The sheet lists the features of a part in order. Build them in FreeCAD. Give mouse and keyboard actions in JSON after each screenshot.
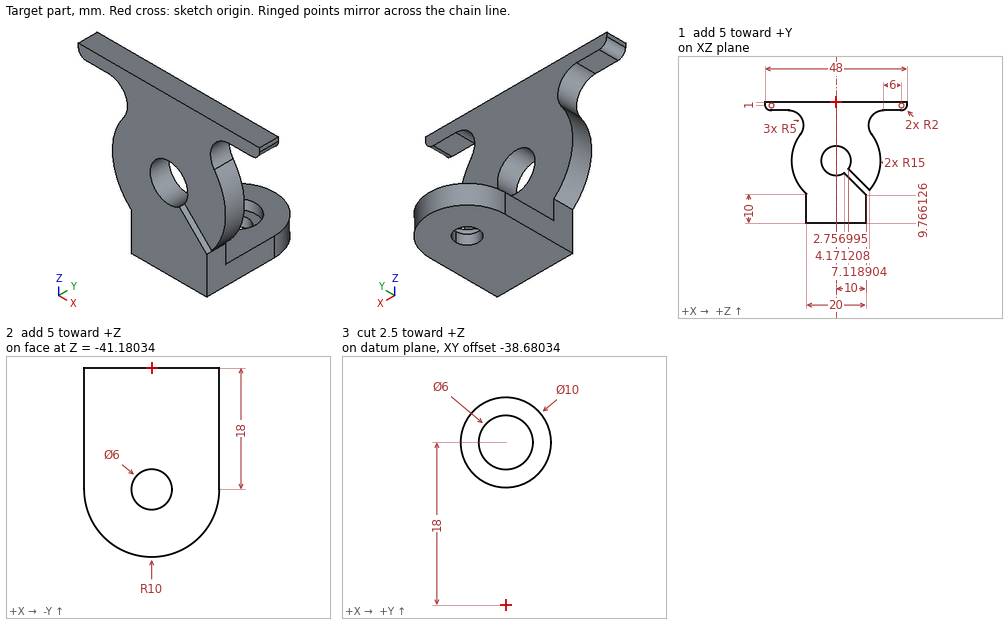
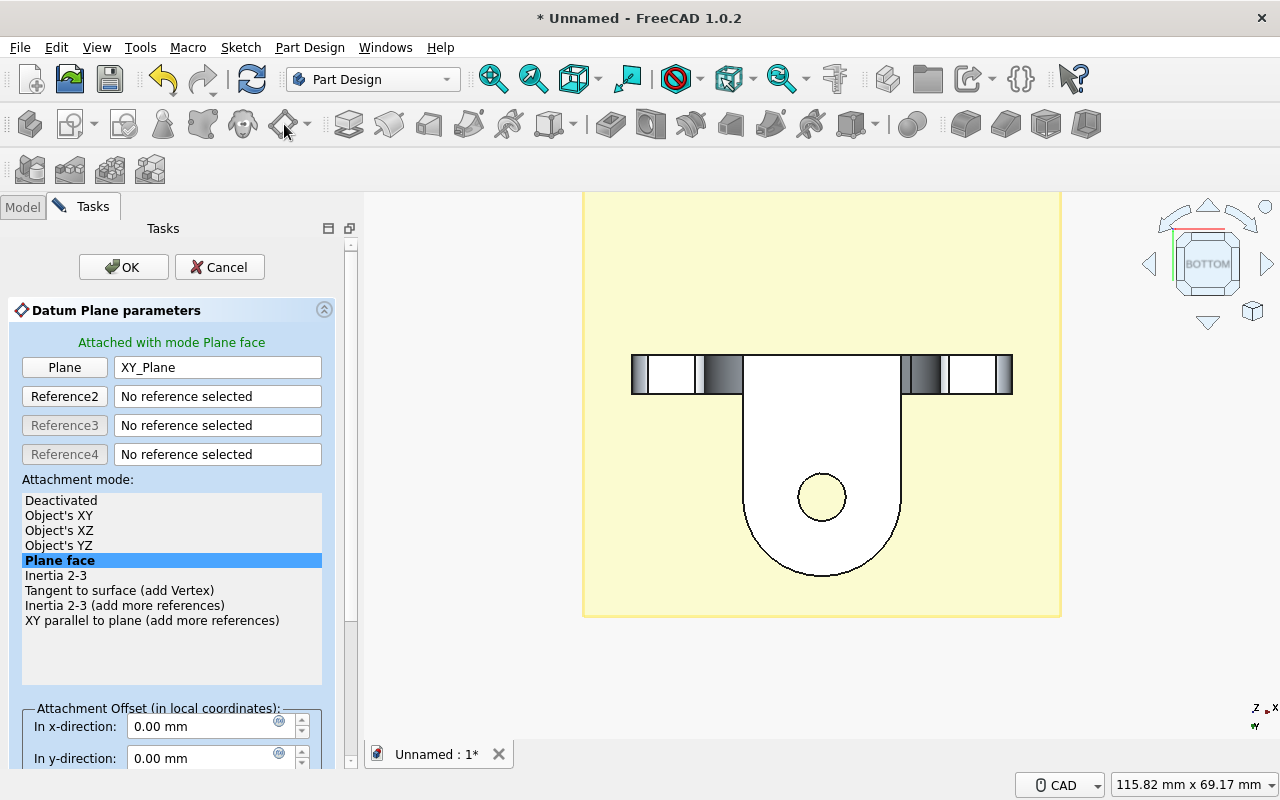
{"action": "scroll", "coordinate": [351, 503], "scroll_direction": "down", "scroll_amount": 2}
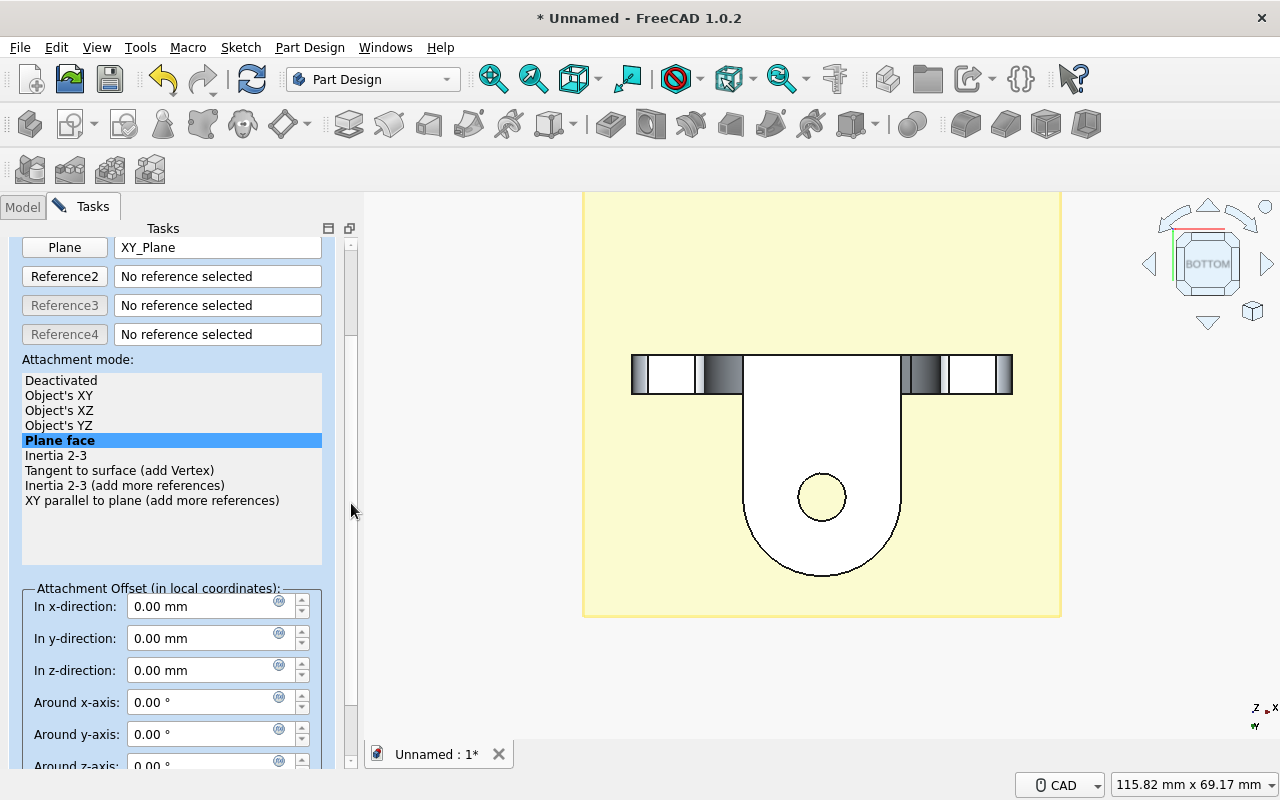
{"action": "triple_click", "coordinate": [210, 670]}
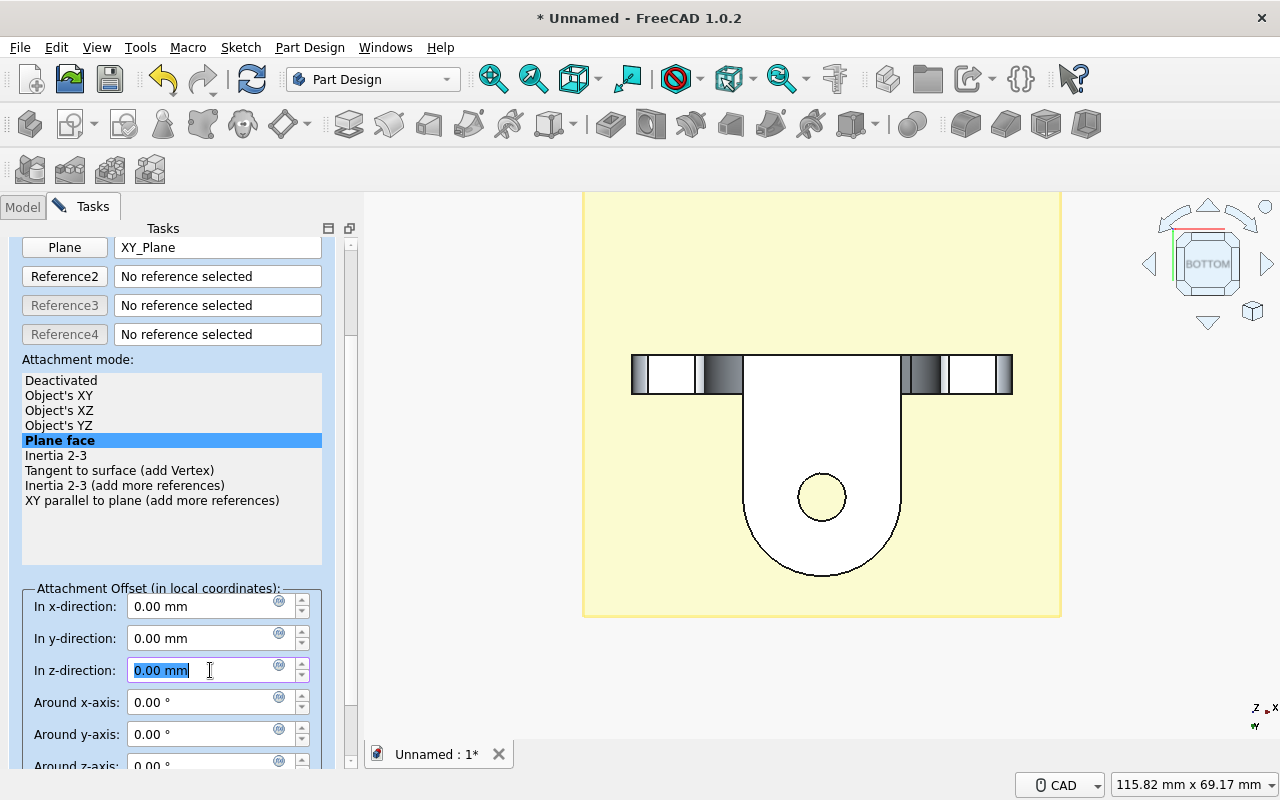
{"action": "type", "text": "-38.68034"}
{"action": "key", "text": "Tab"}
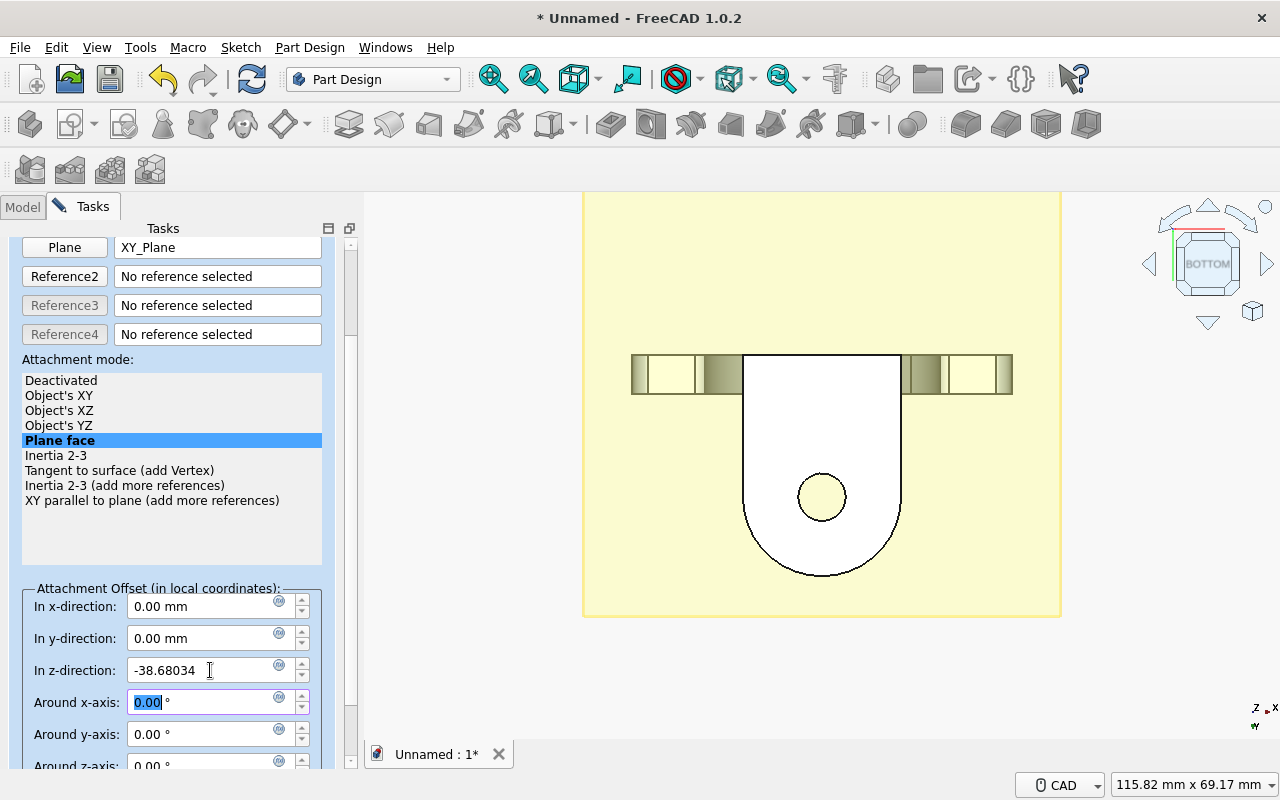
{"action": "scroll", "coordinate": [351, 503], "scroll_direction": "up", "scroll_amount": 3}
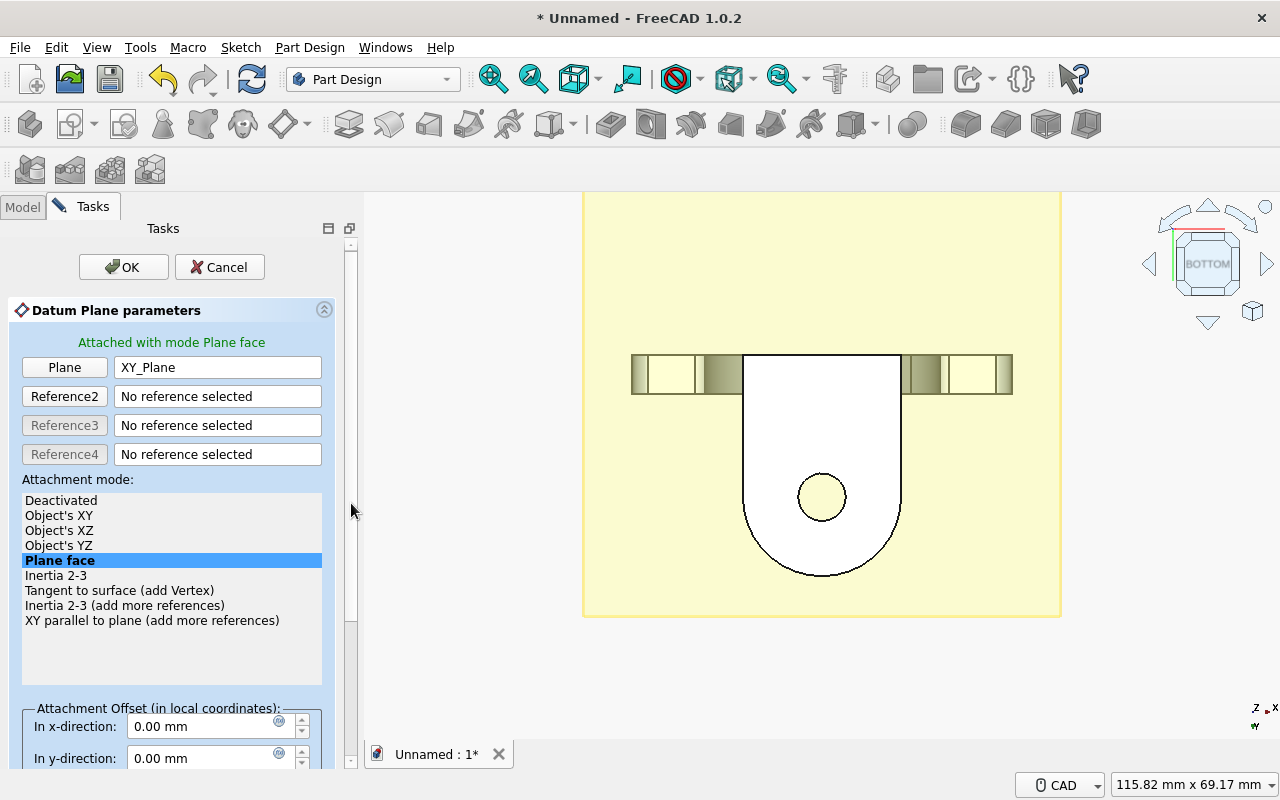
{"action": "left_click", "coordinate": [124, 267]}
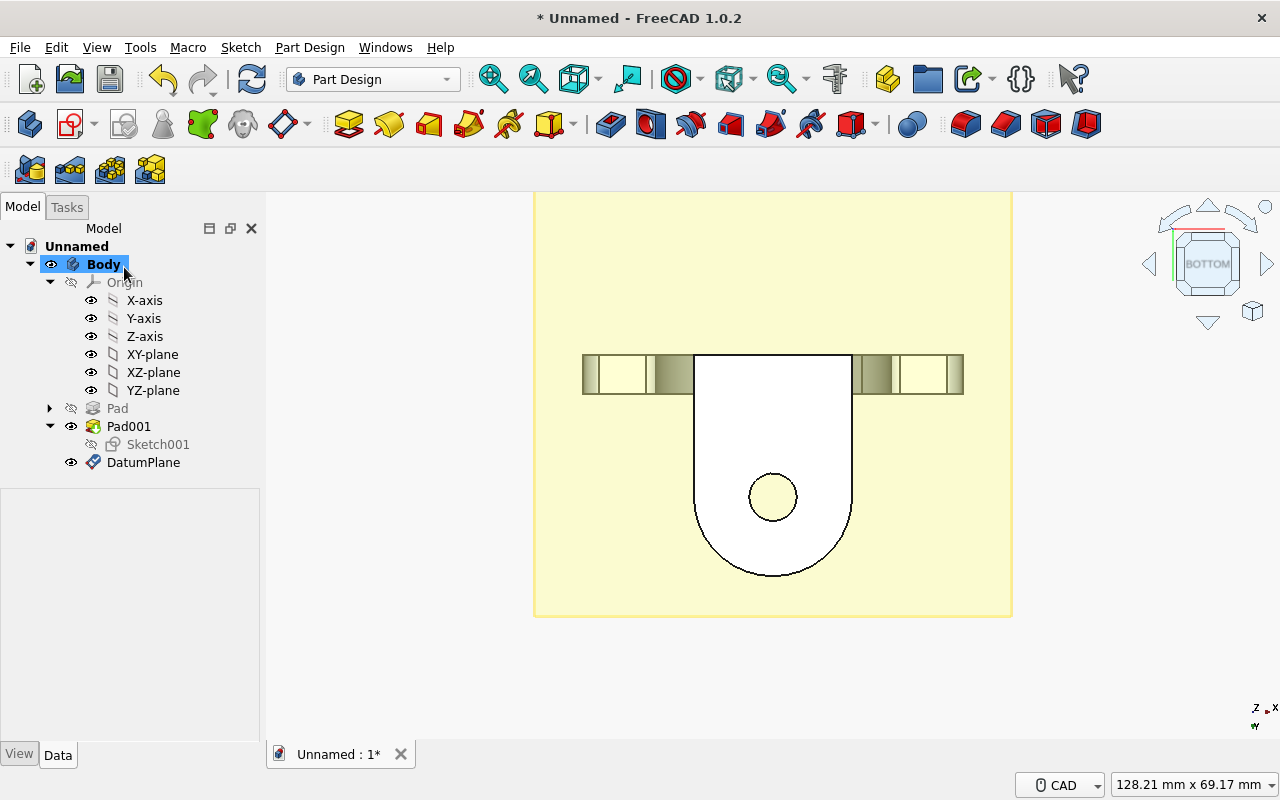
{"action": "left_click", "coordinate": [116, 462]}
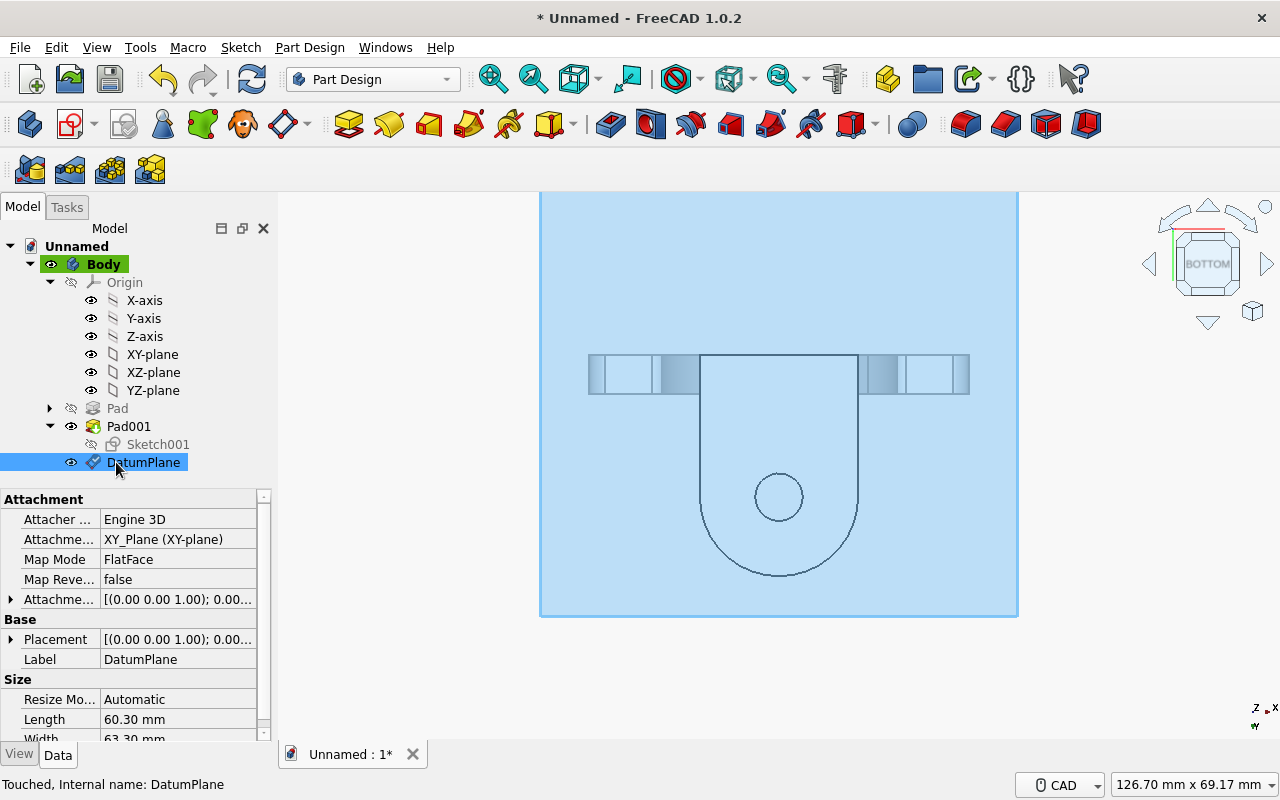
{"action": "left_click", "coordinate": [70, 124]}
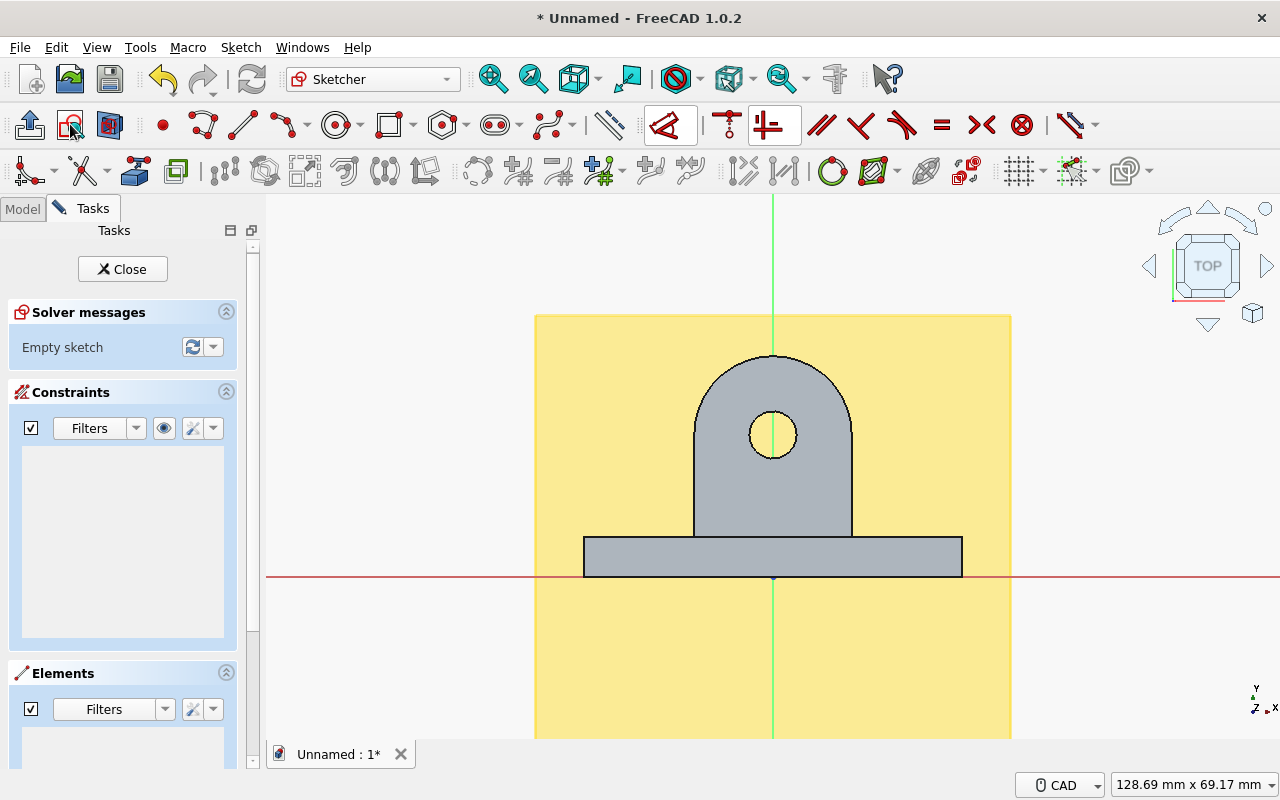
{"action": "key", "text": "q s"}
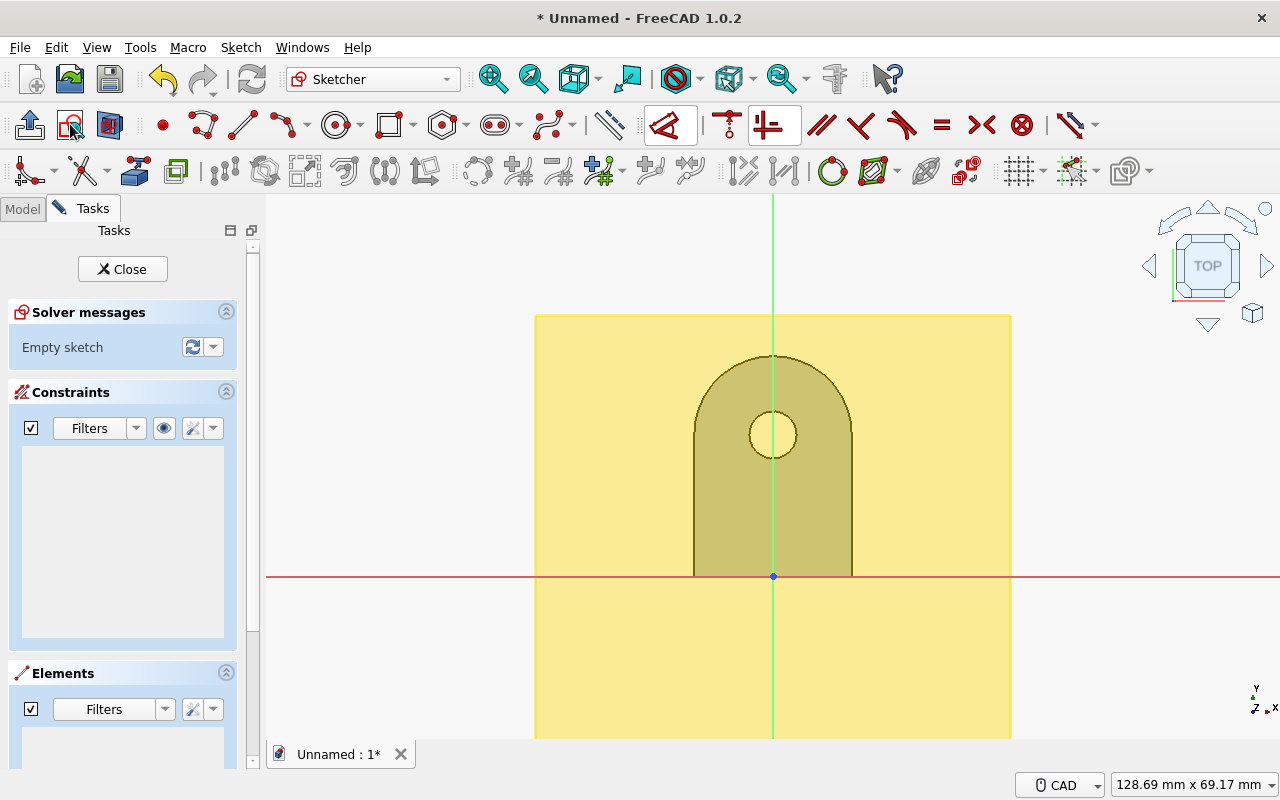
{"action": "scroll", "coordinate": [856, 510], "scroll_direction": "up", "scroll_amount": 3}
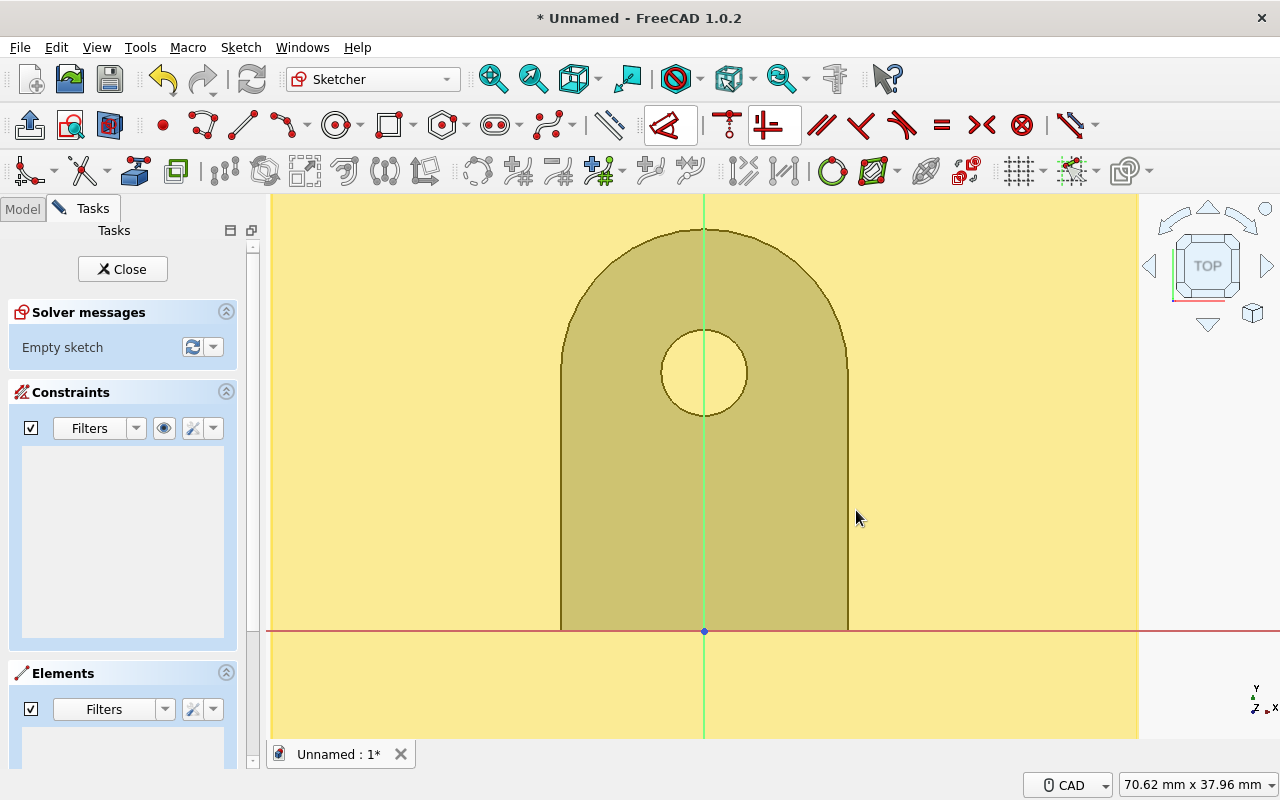
{"action": "key", "text": "g c"}